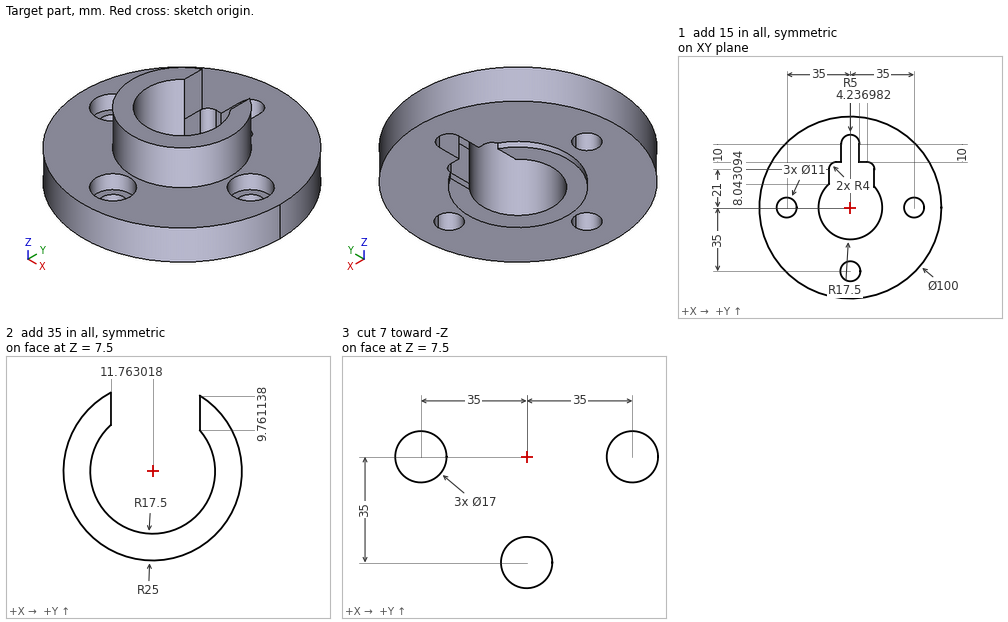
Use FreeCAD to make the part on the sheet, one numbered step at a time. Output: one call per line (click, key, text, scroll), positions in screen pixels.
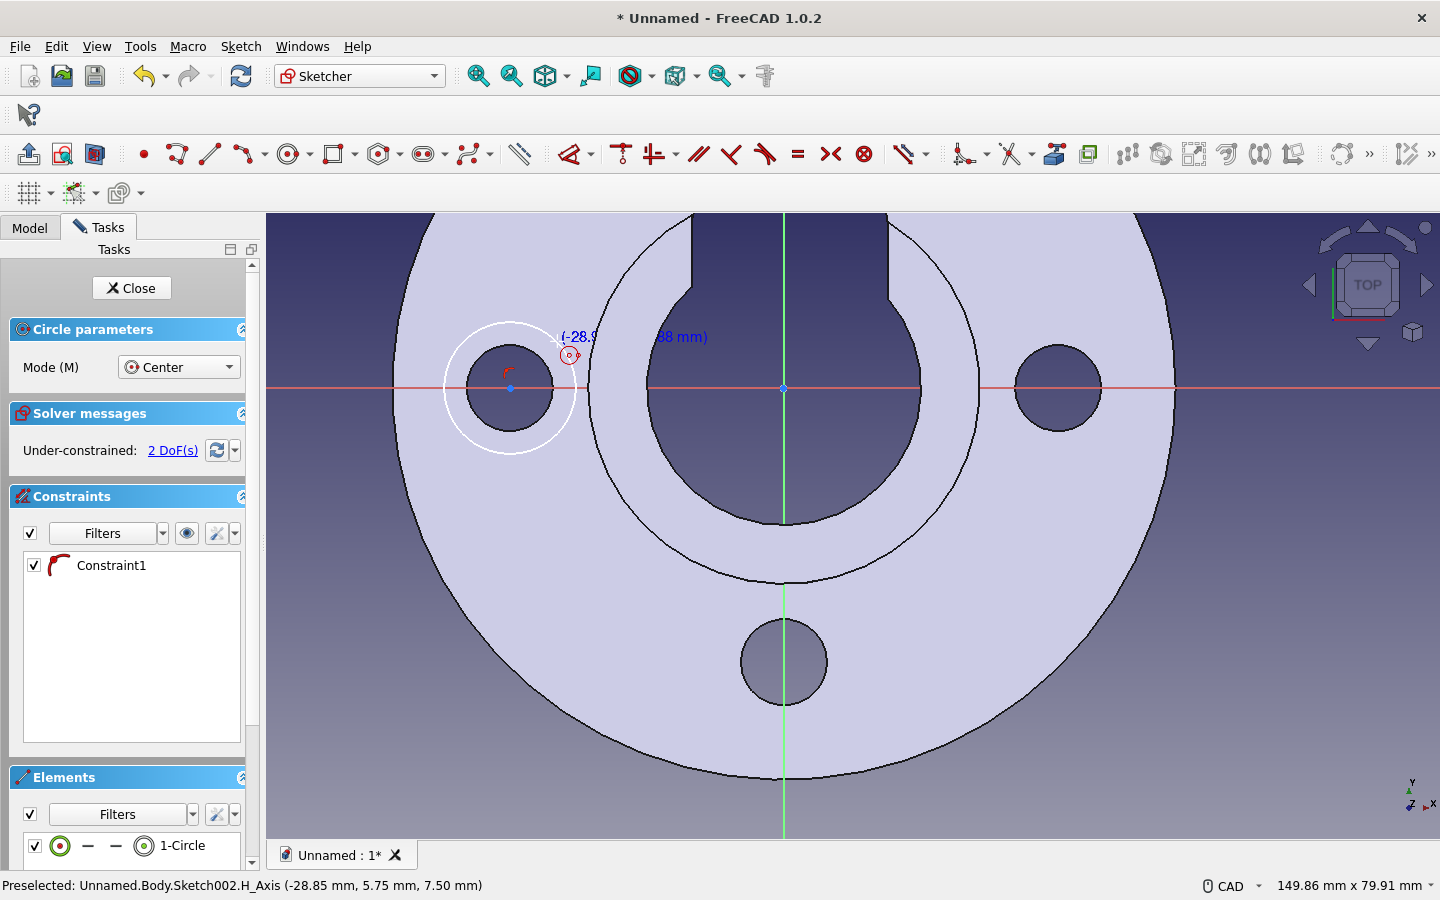
click(1058, 388)
click(1105, 341)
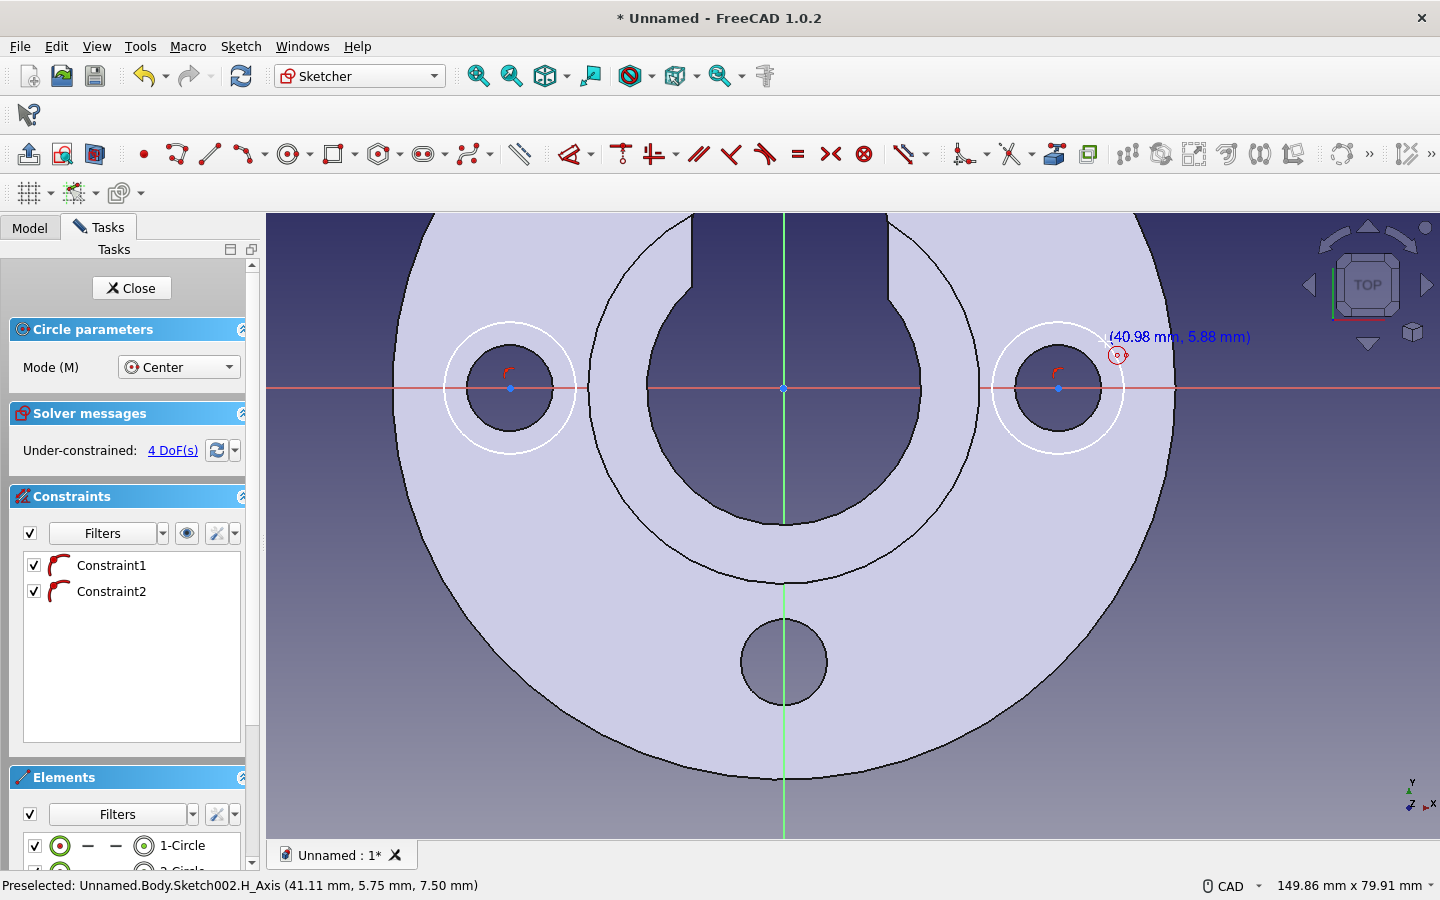
click(784, 662)
click(831, 615)
key(Escape)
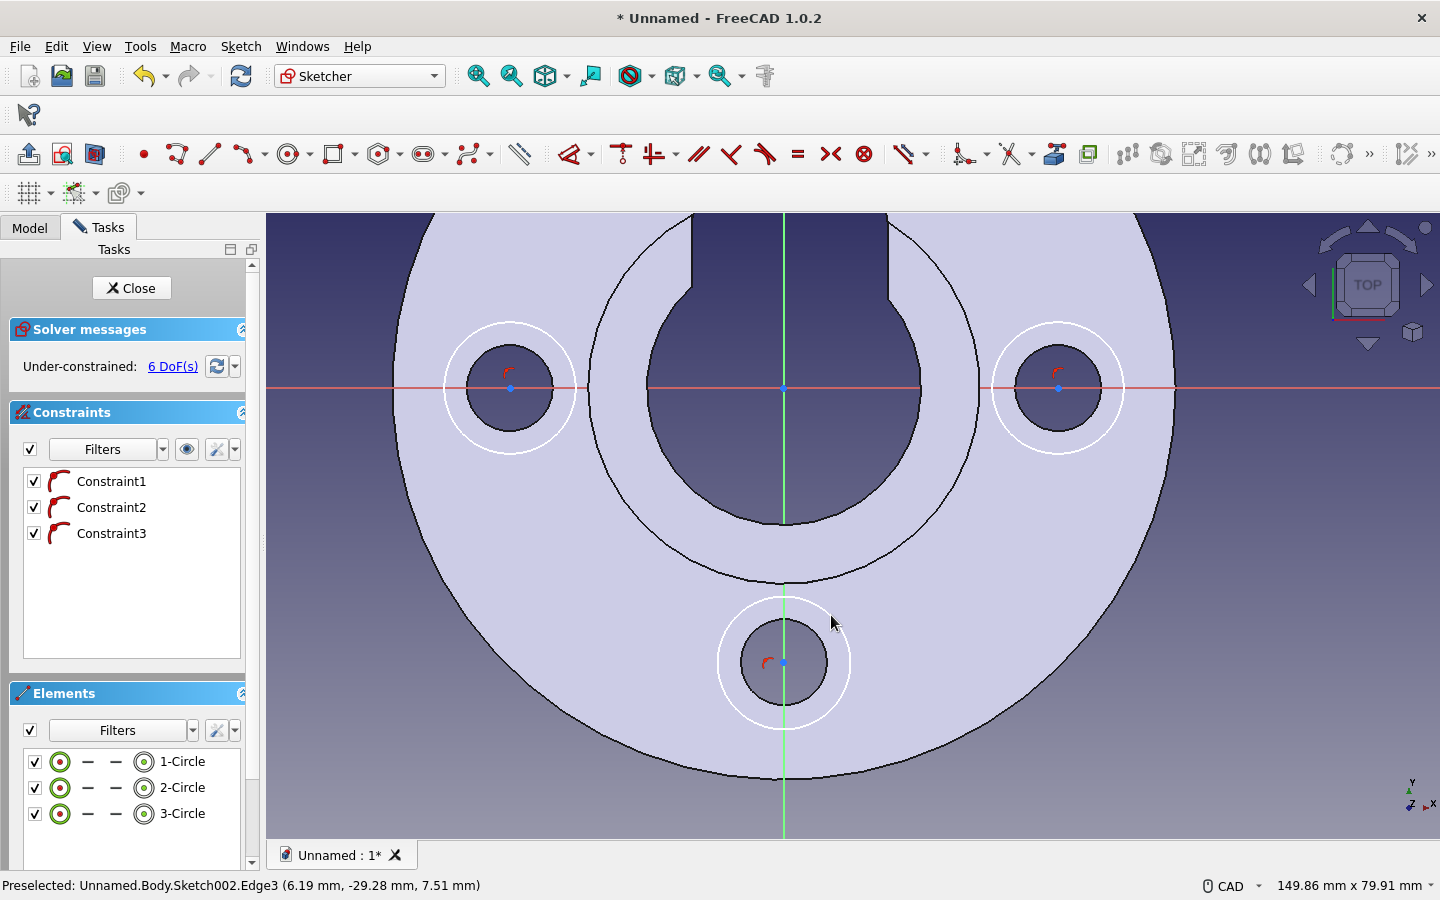
click(556, 341)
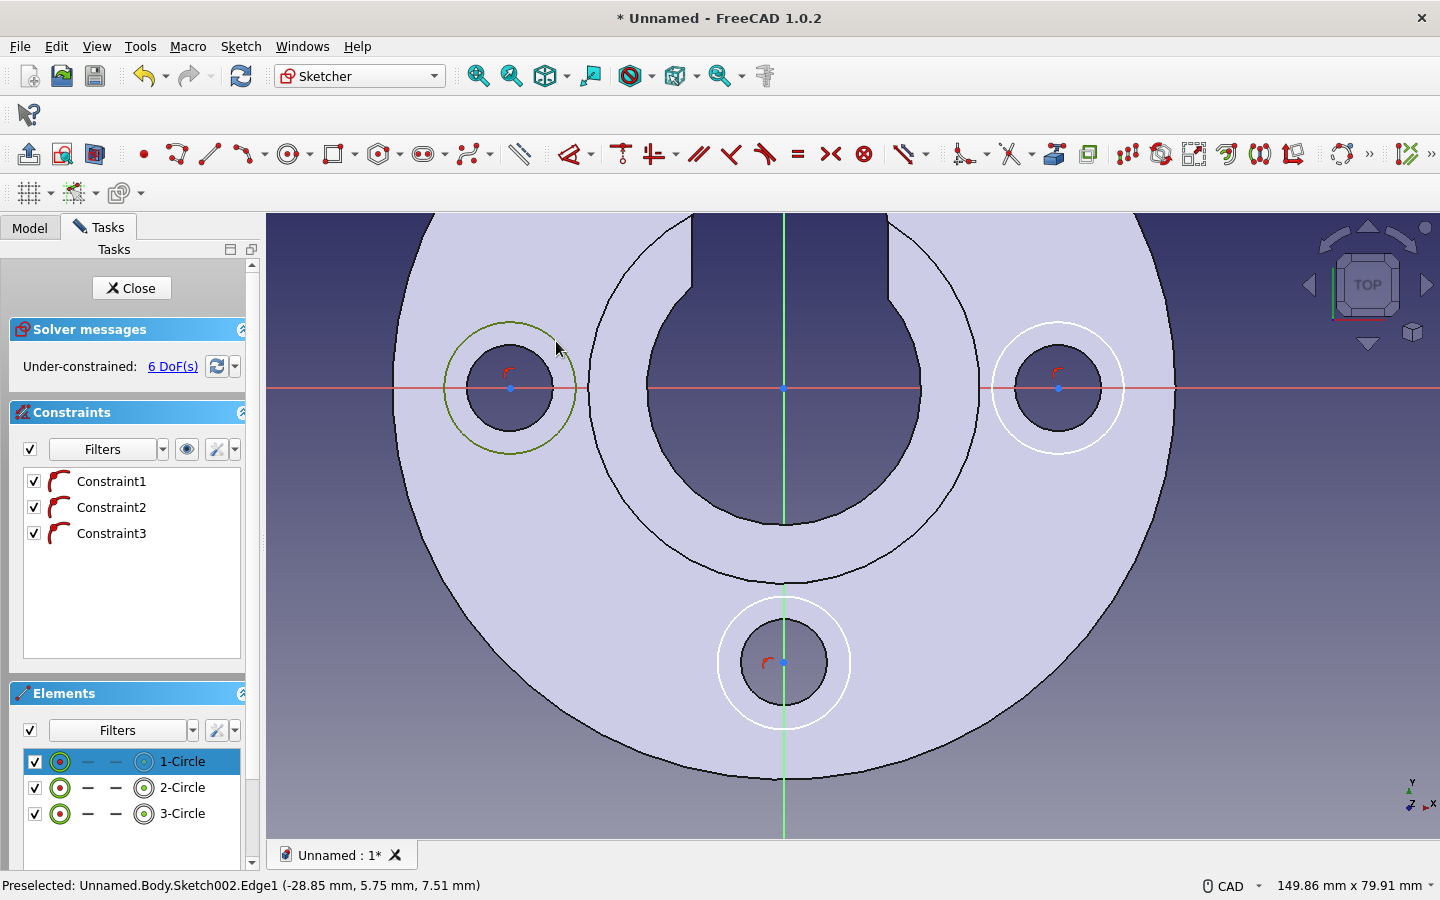
click(1104, 341)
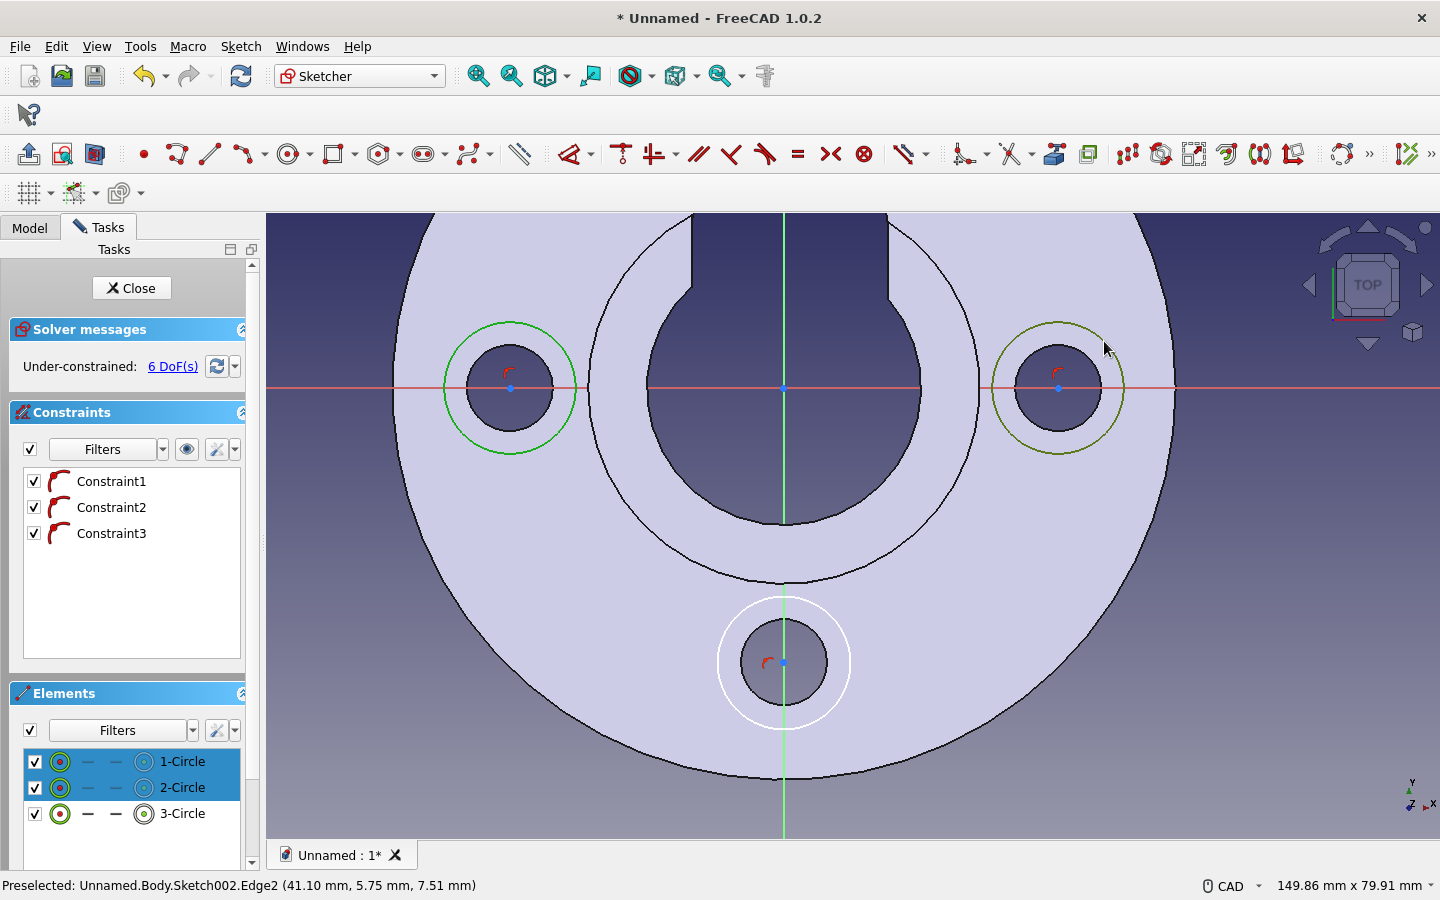
click(831, 616)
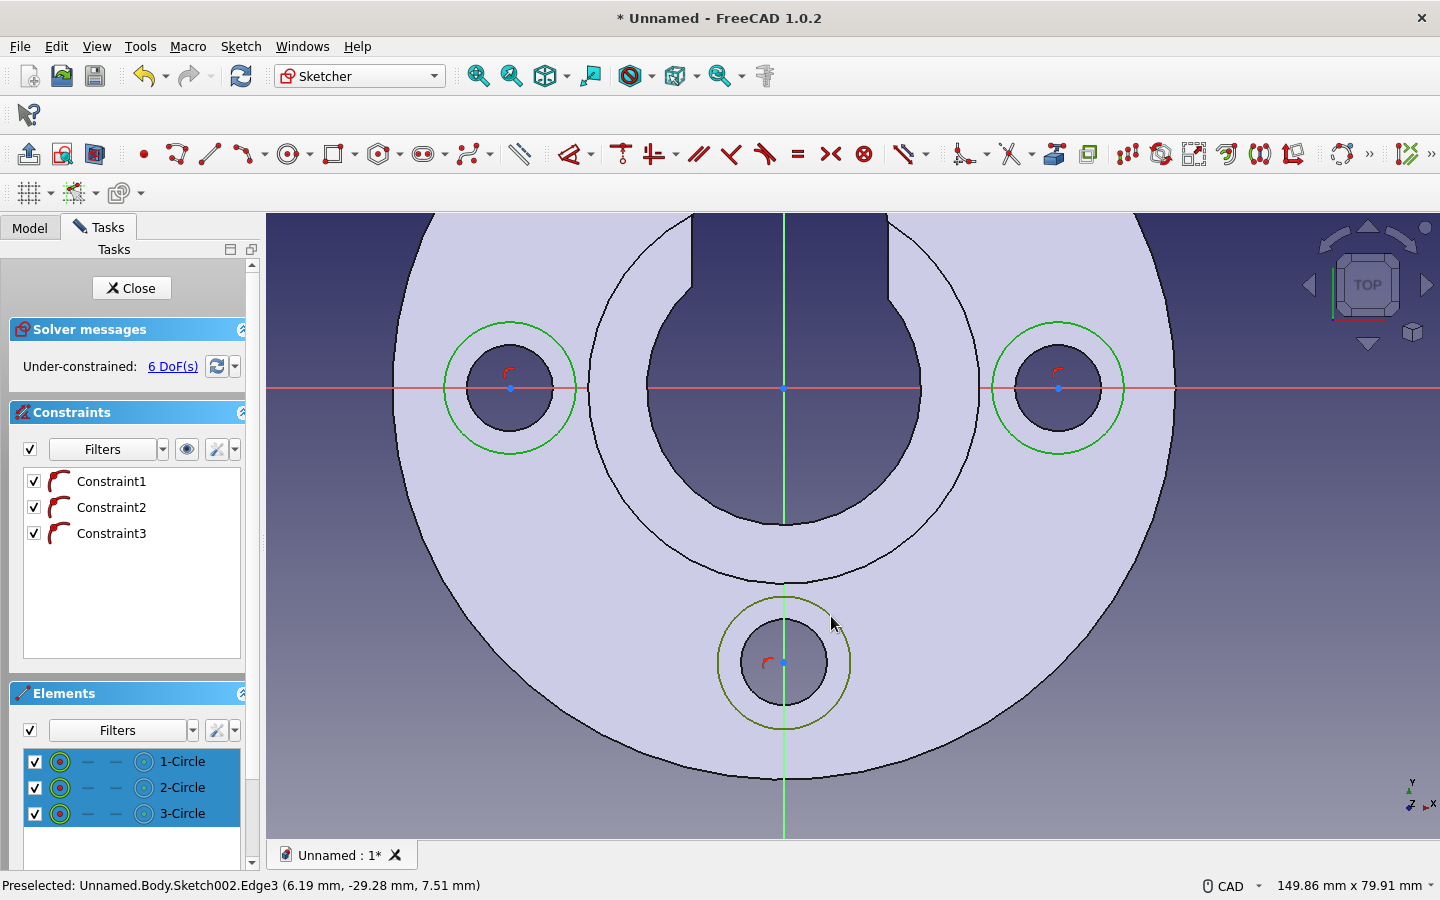
key(e)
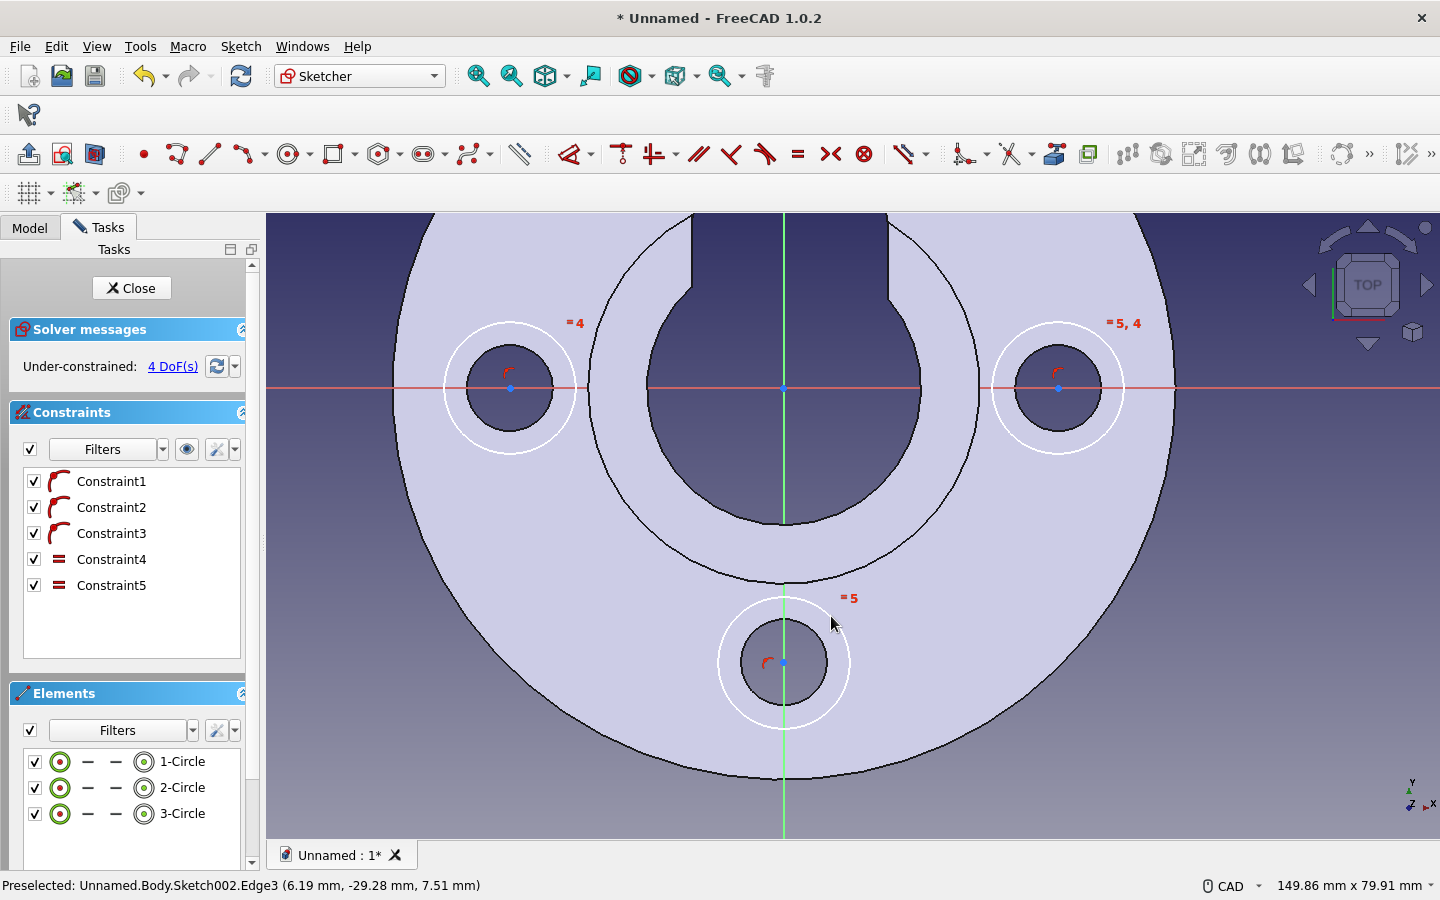
click(568, 154)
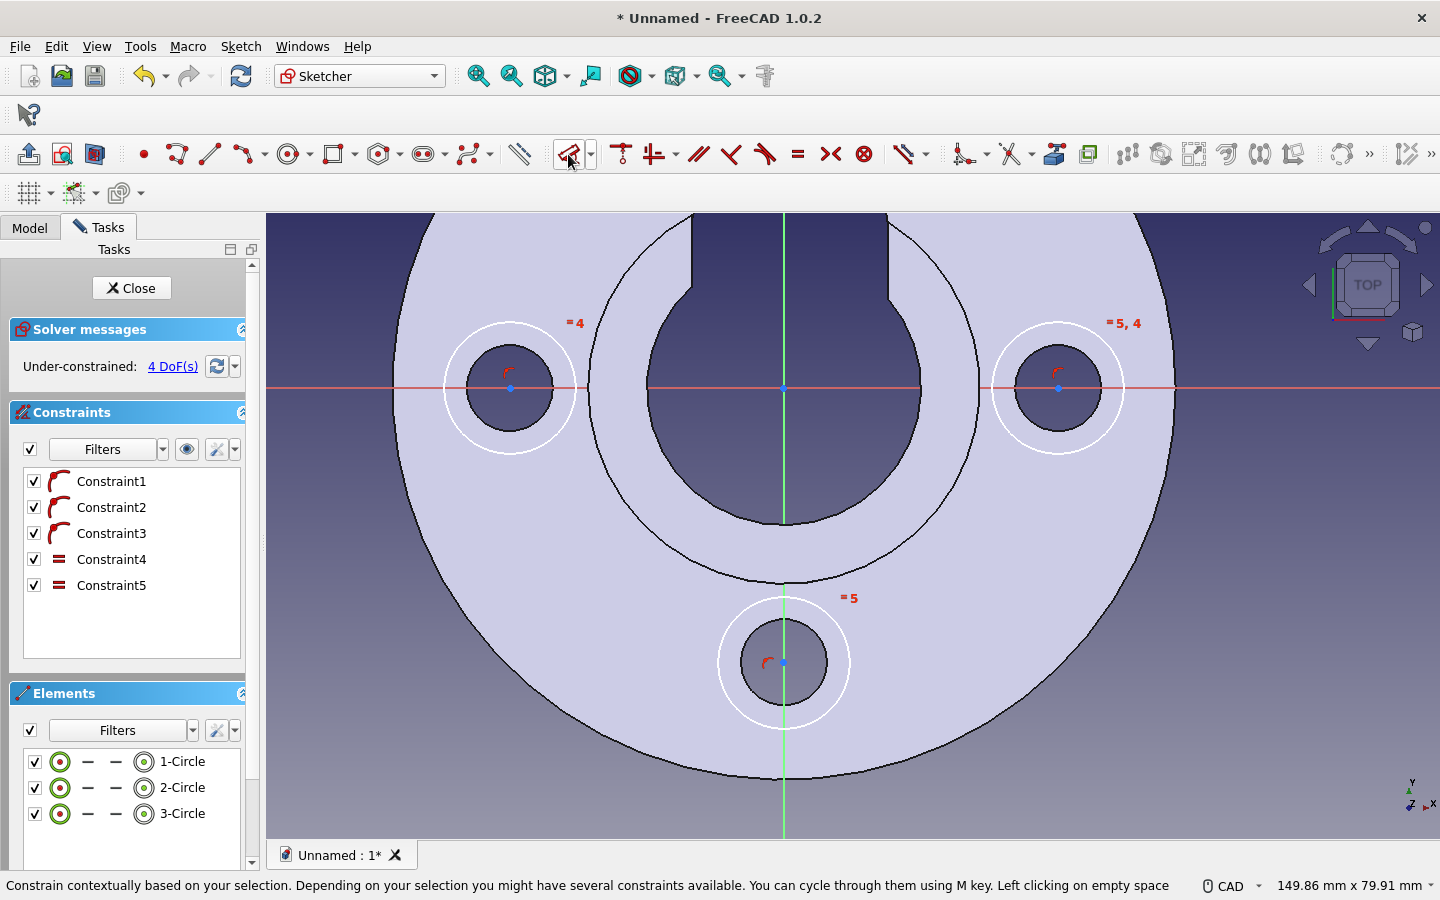
click(556, 341)
click(578, 318)